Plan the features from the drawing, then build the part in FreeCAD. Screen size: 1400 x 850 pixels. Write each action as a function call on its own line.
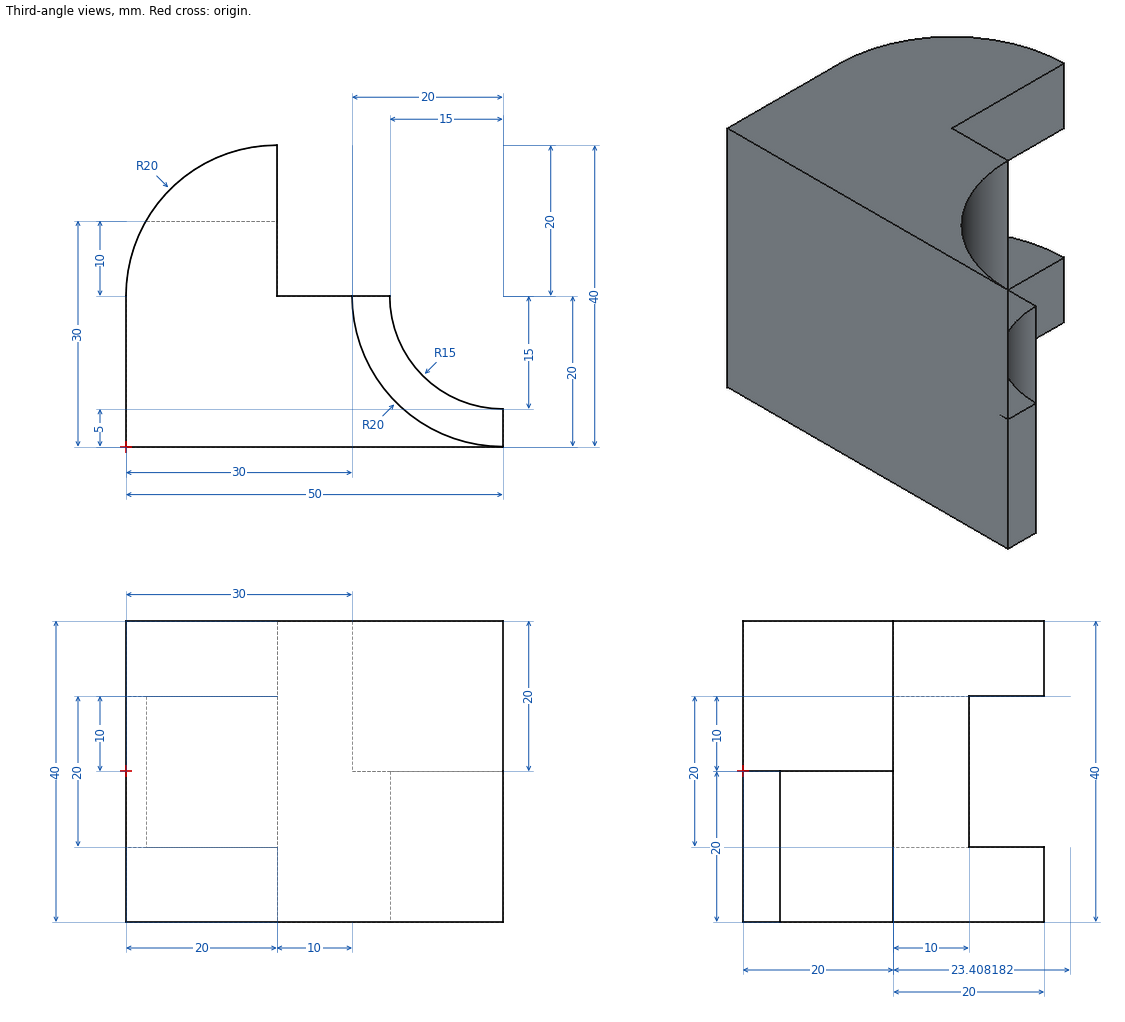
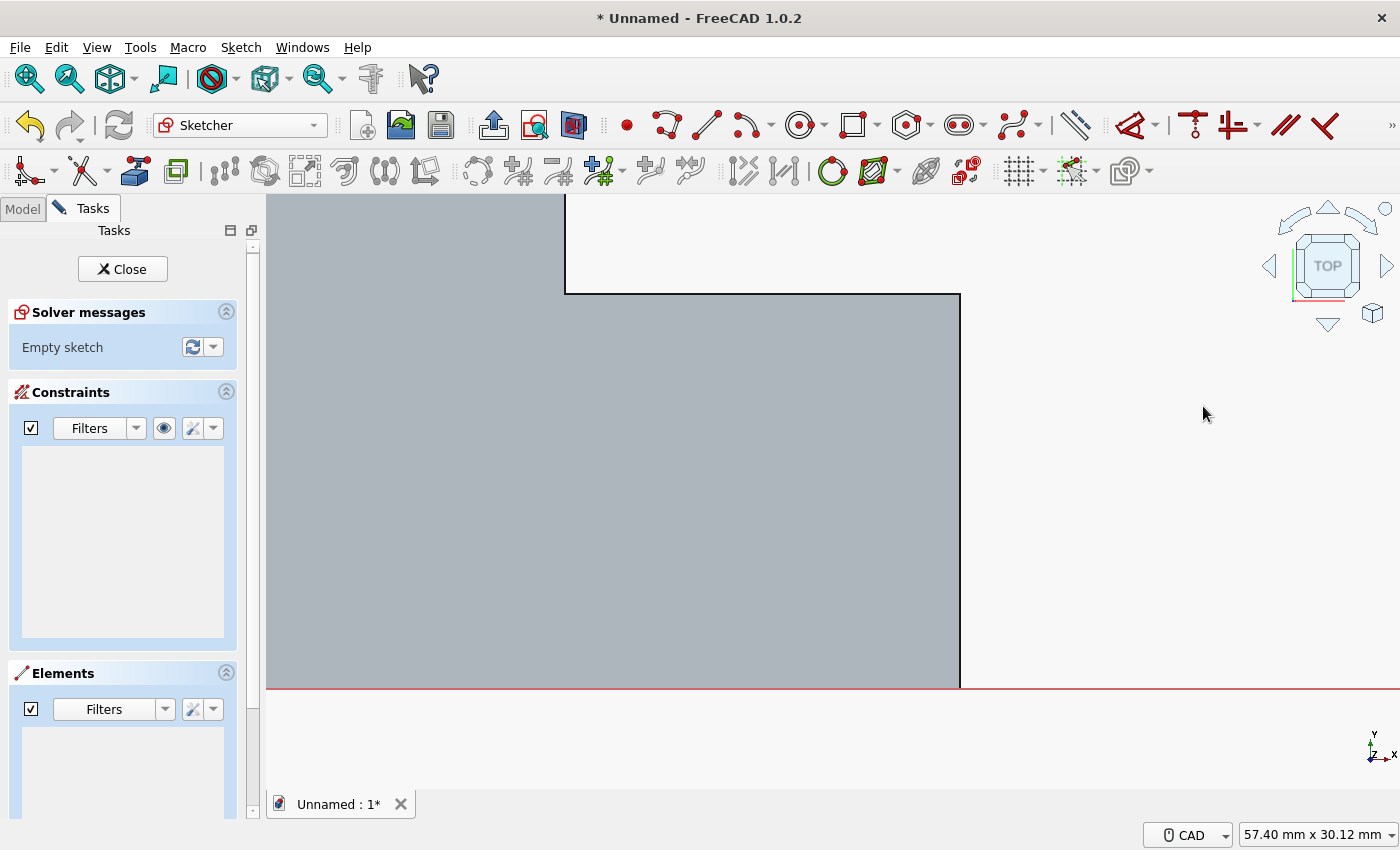
click(668, 126)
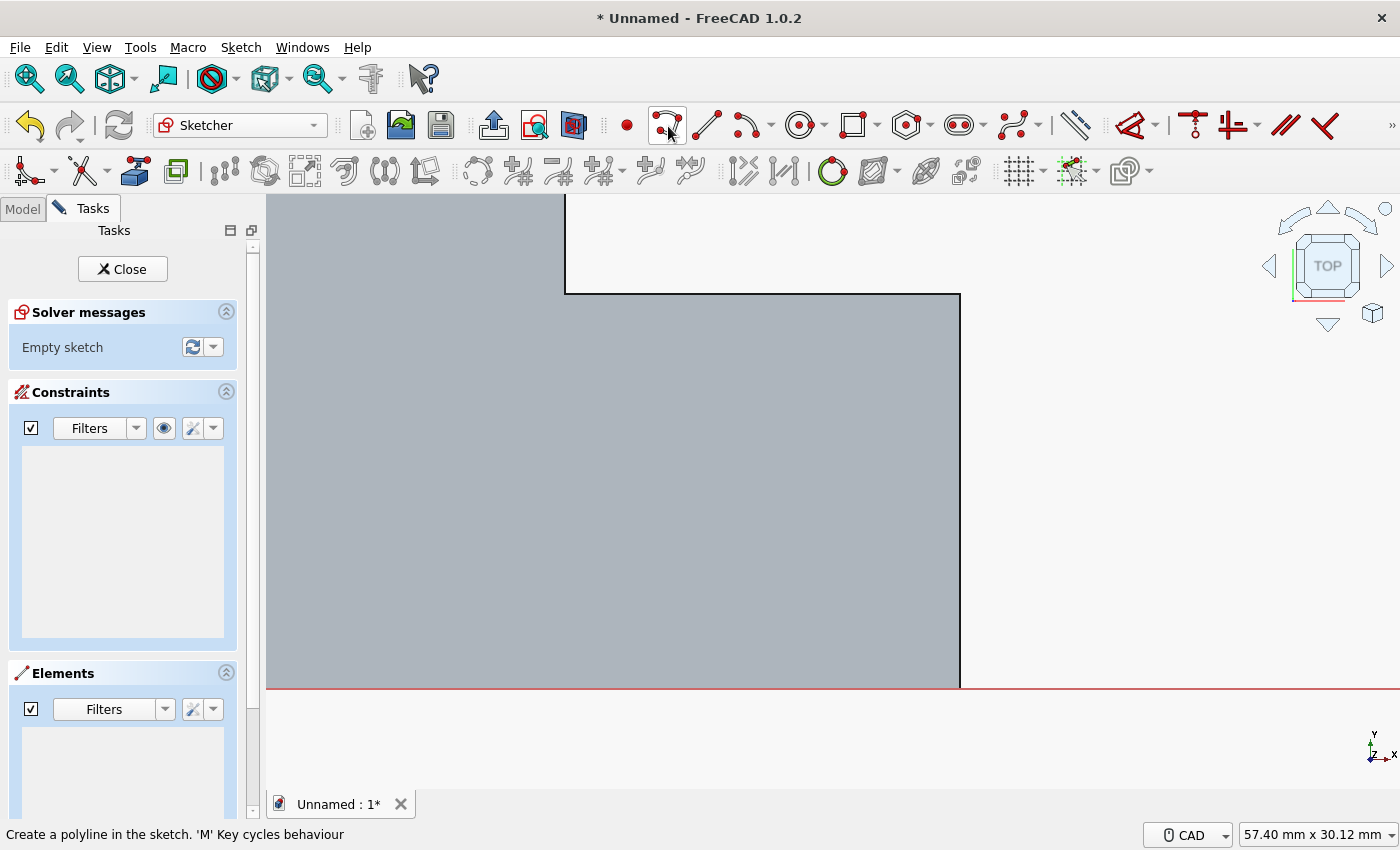
click(960, 689)
click(960, 294)
click(565, 294)
right_click(565, 294)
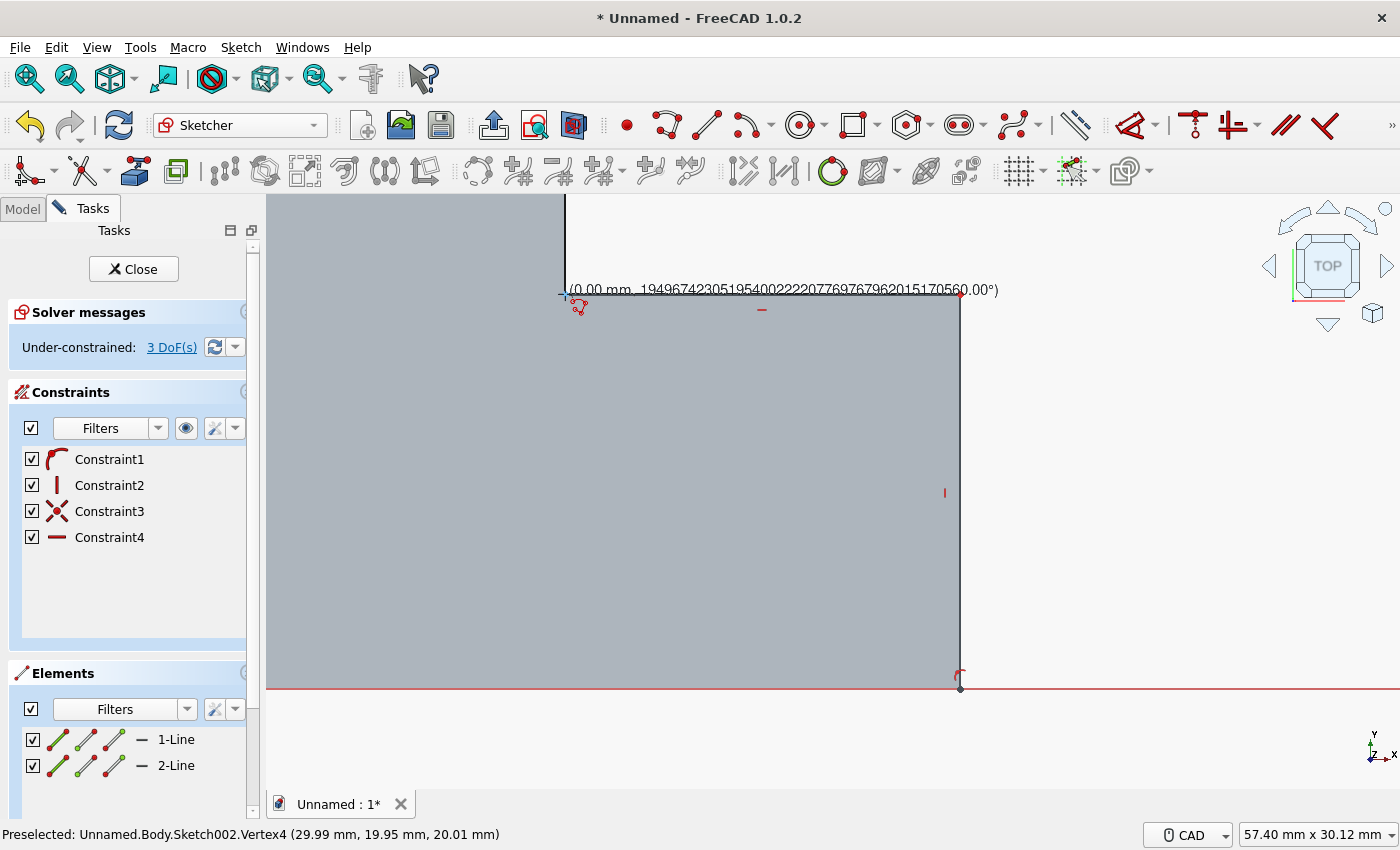
key(g)
key(3)
key(a)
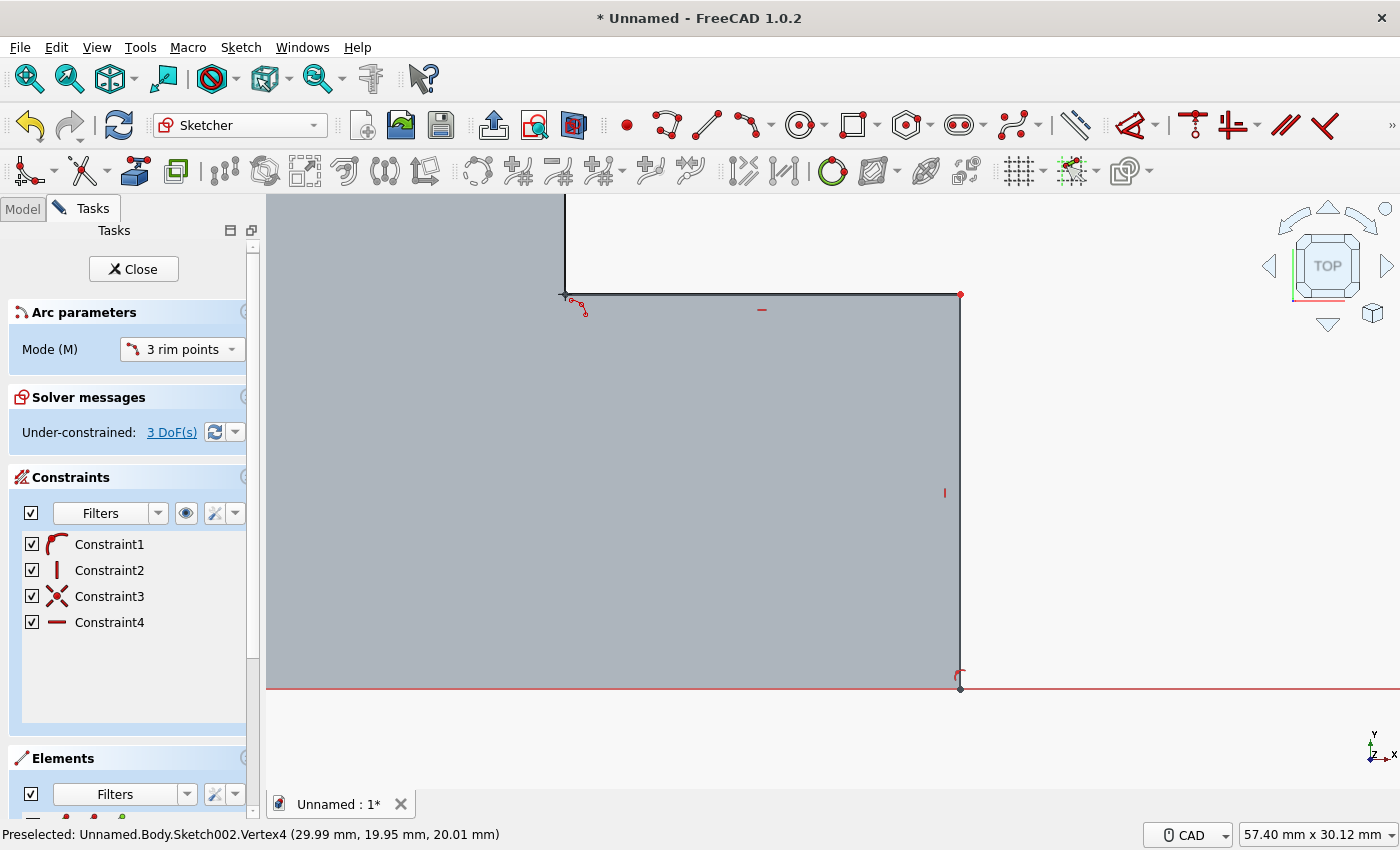
click(565, 295)
click(960, 689)
click(681, 573)
key(Escape)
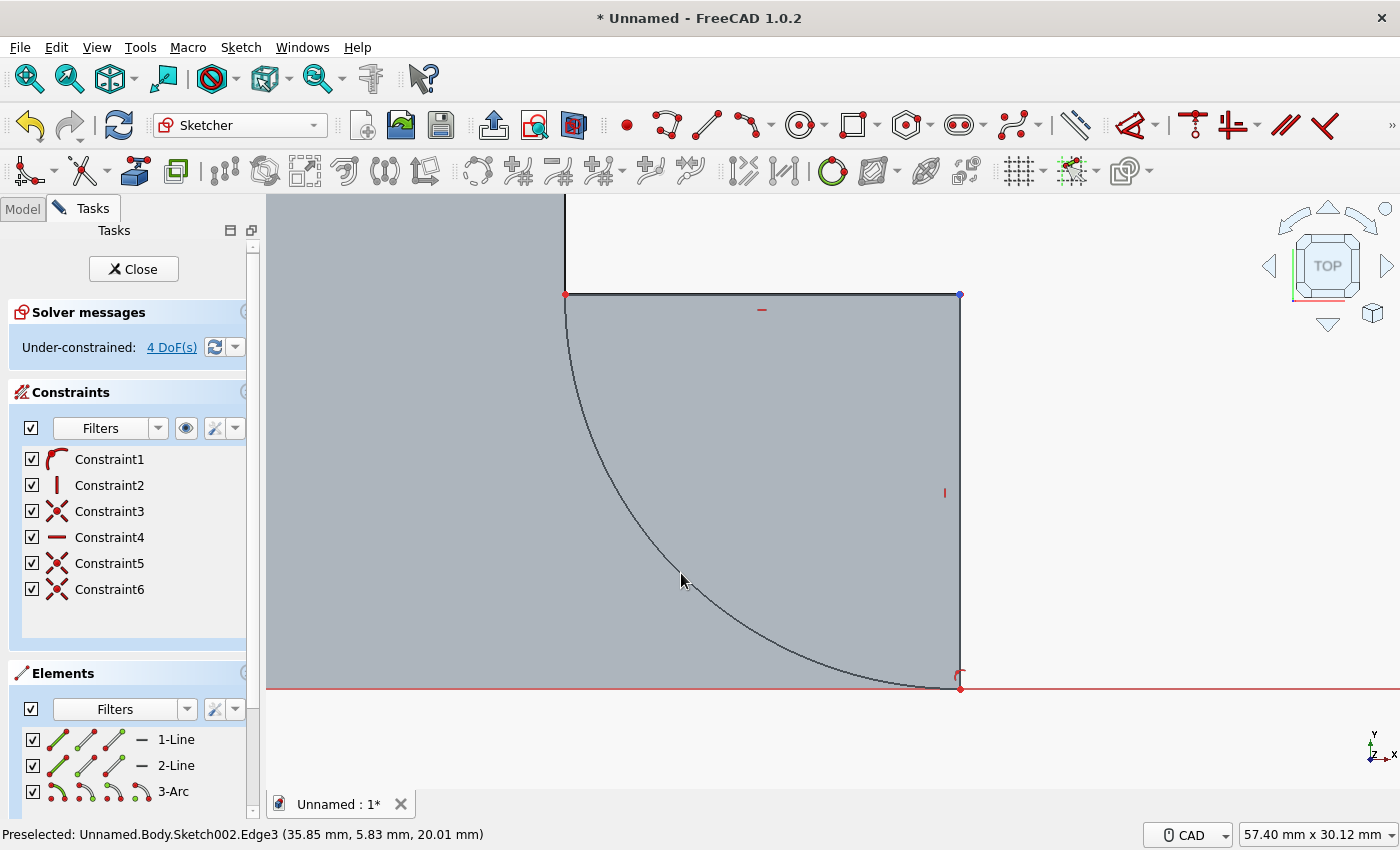
click(1130, 126)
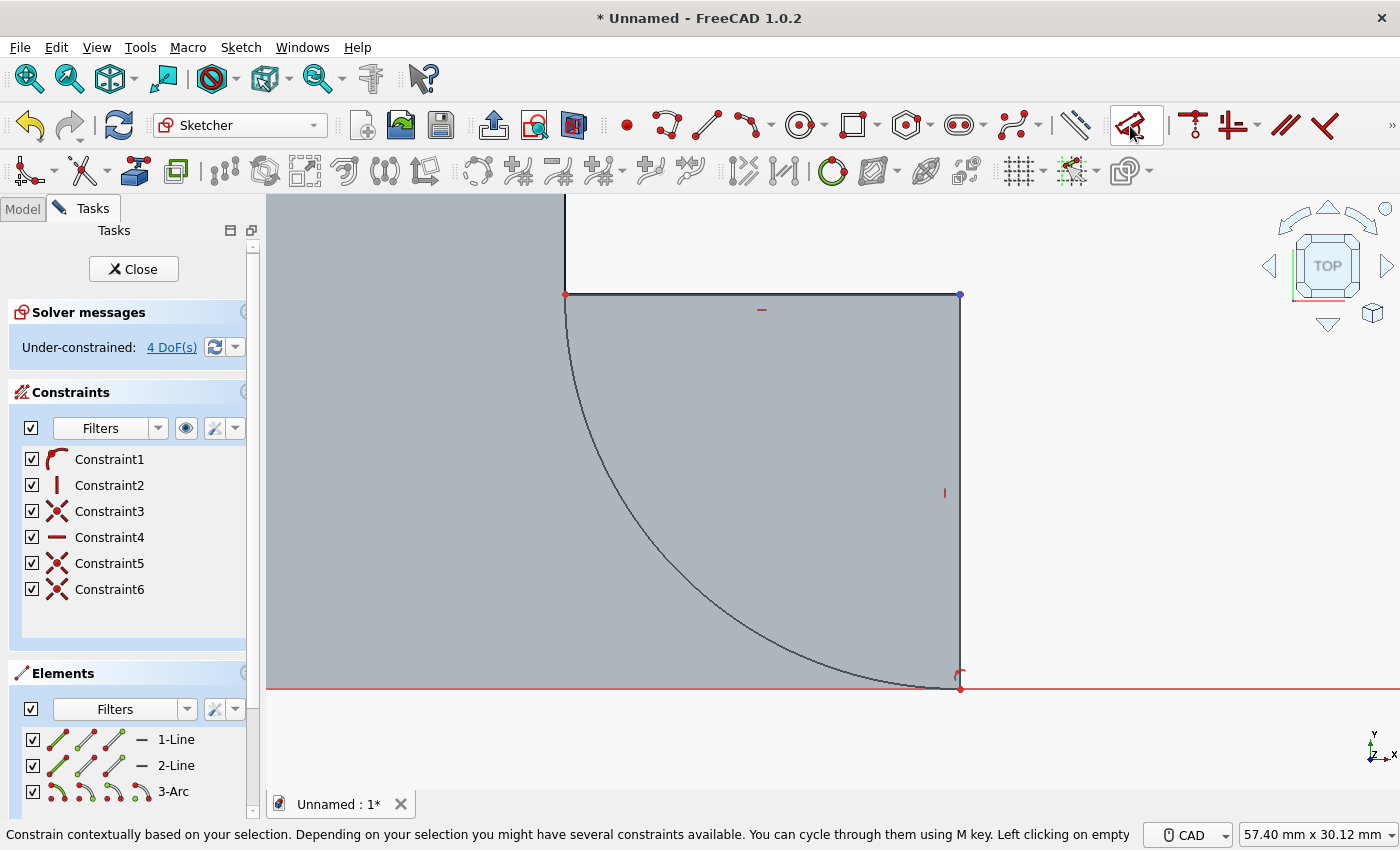
click(608, 474)
click(579, 489)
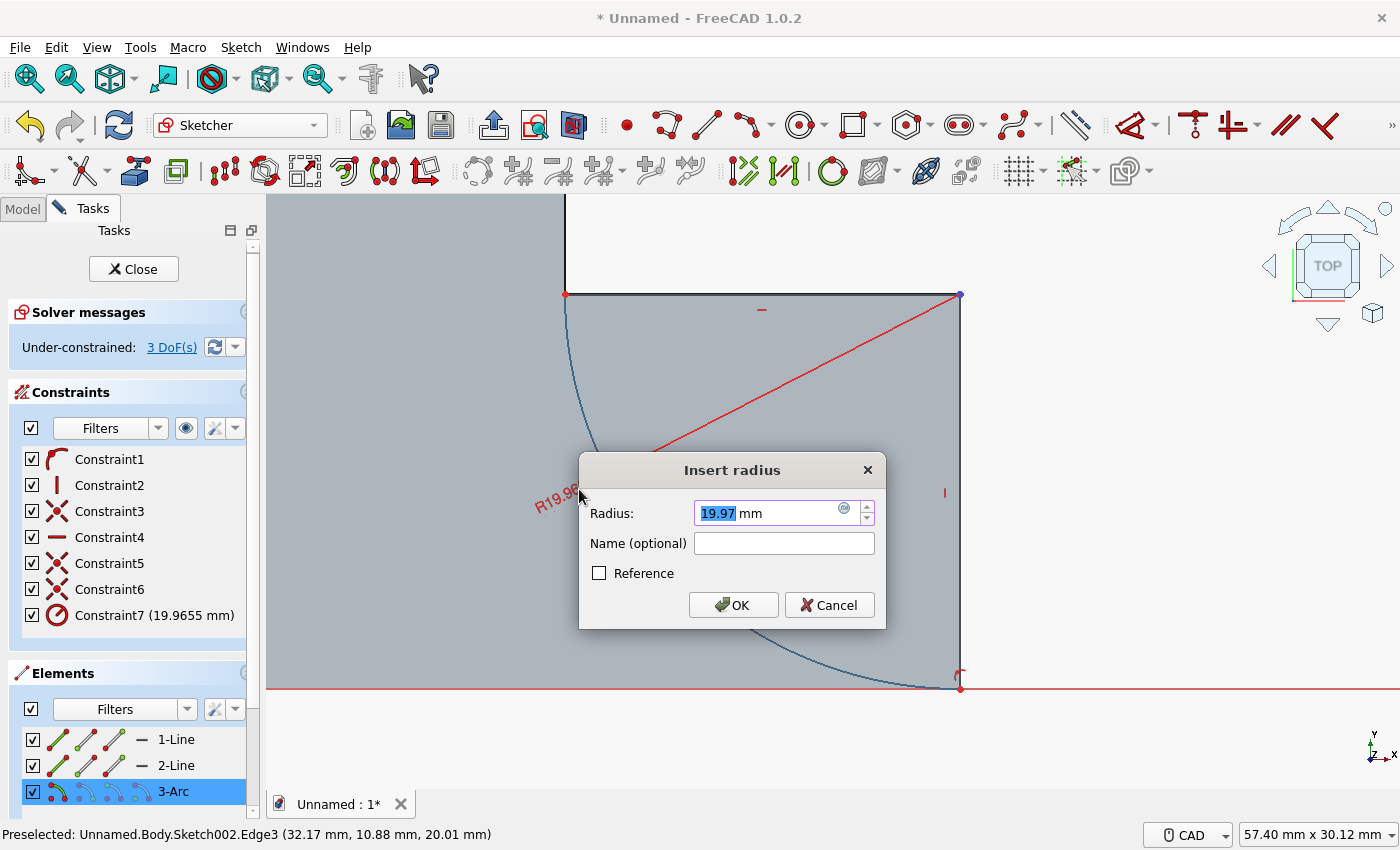
text(20)
key(Return)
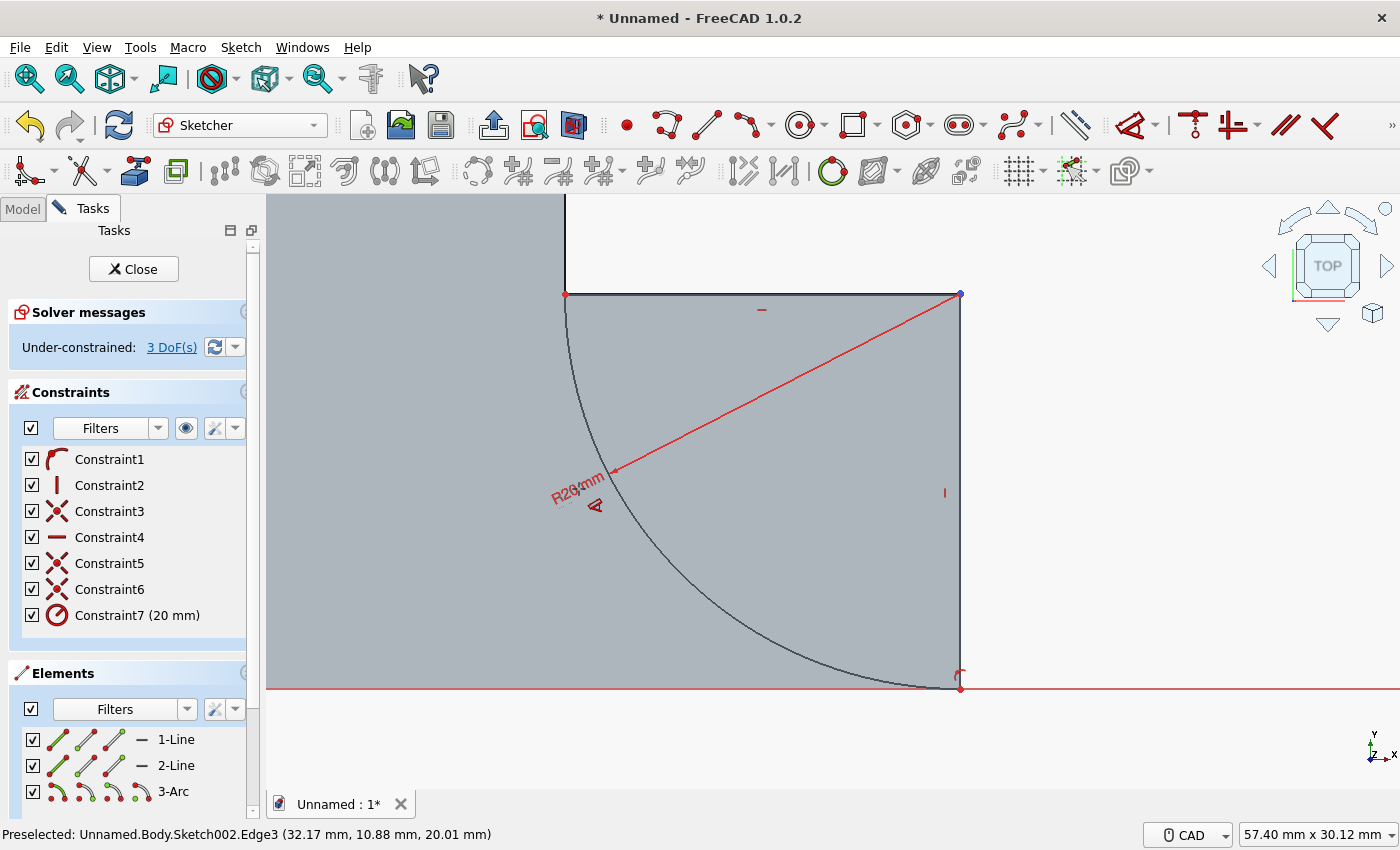
click(960, 571)
click(994, 492)